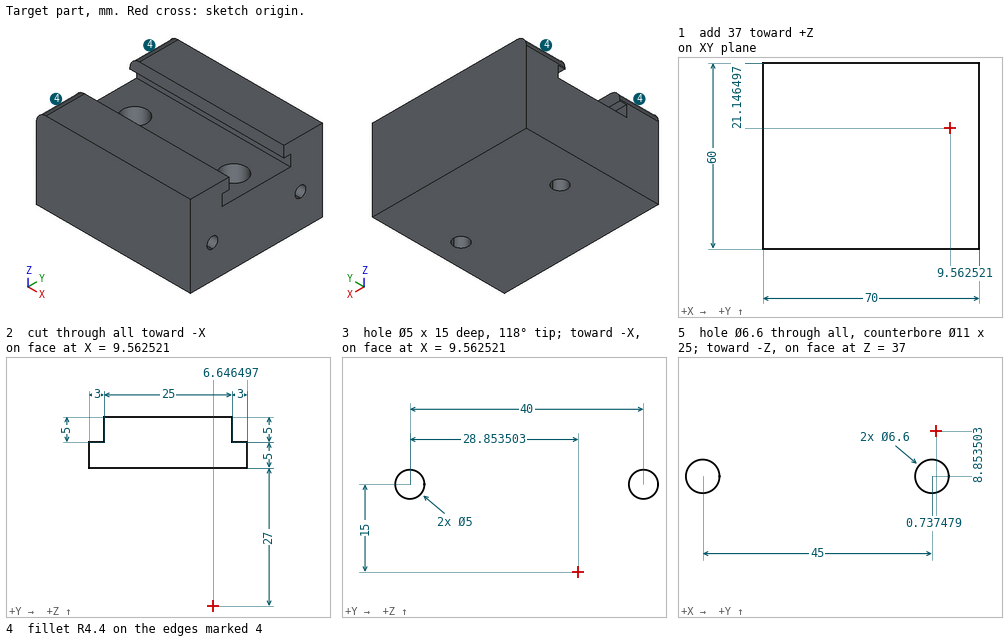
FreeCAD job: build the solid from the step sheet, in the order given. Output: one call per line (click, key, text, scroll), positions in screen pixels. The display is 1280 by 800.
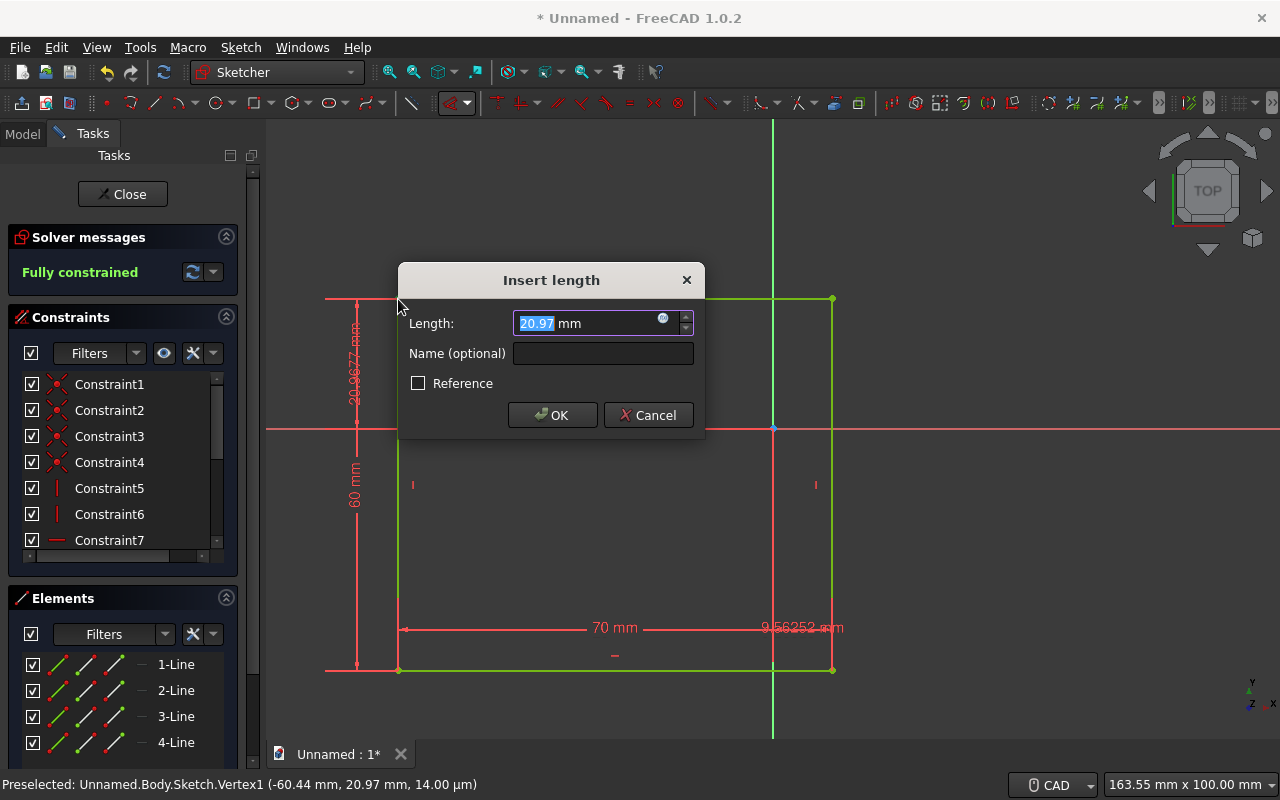
text(21.146497)
key(Return)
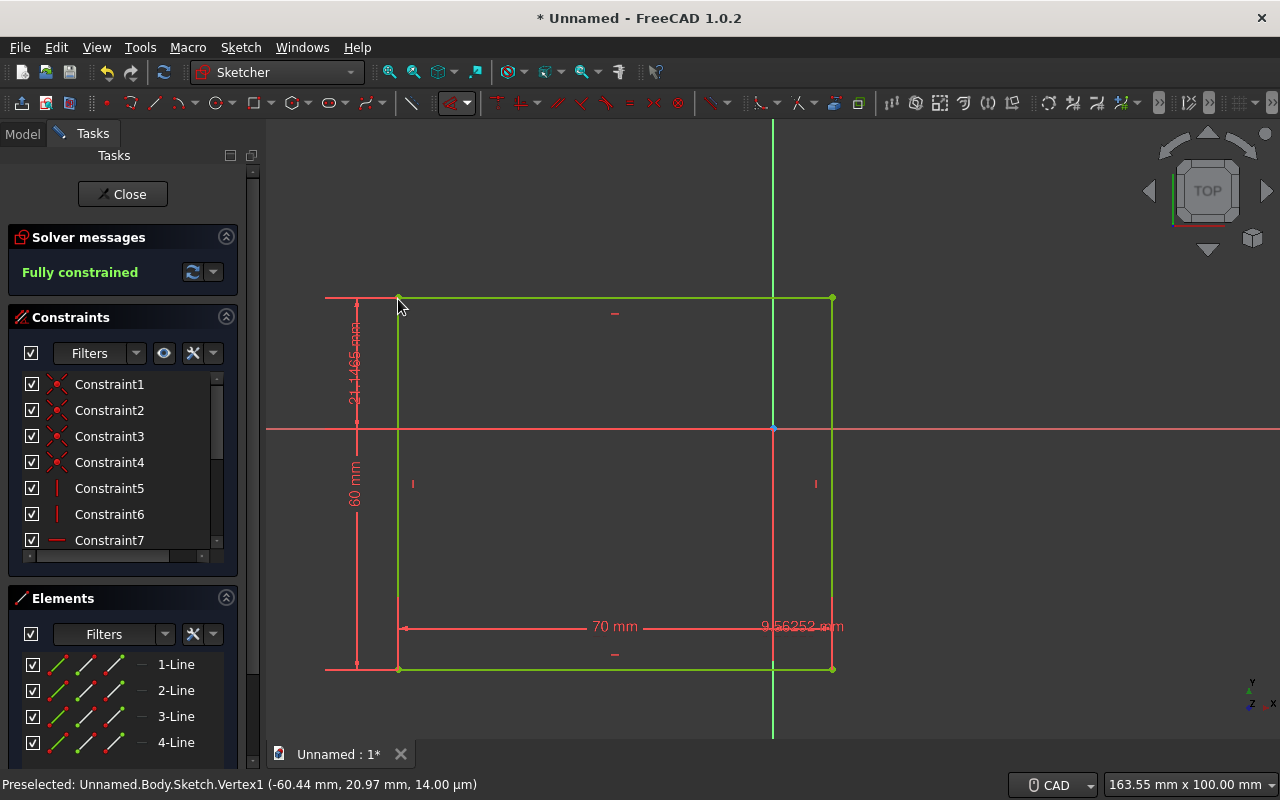
click(123, 194)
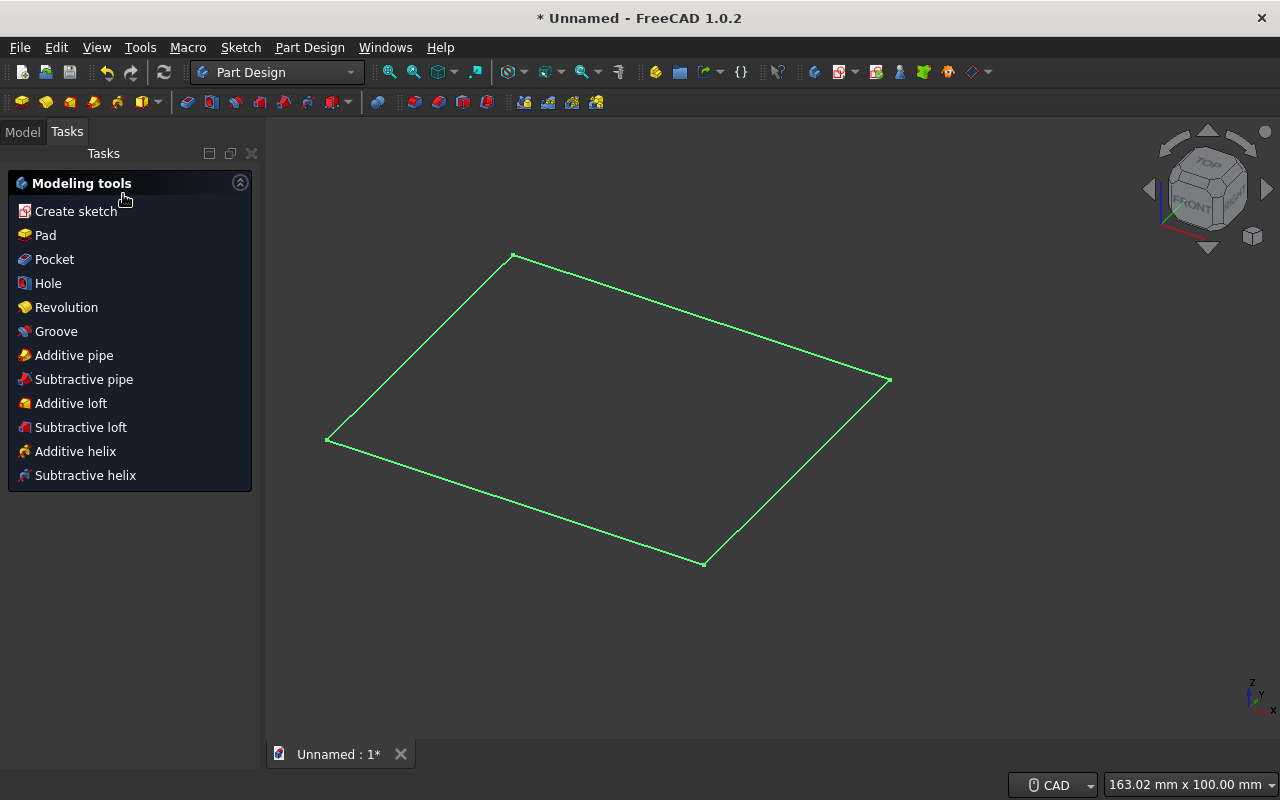
click(22, 102)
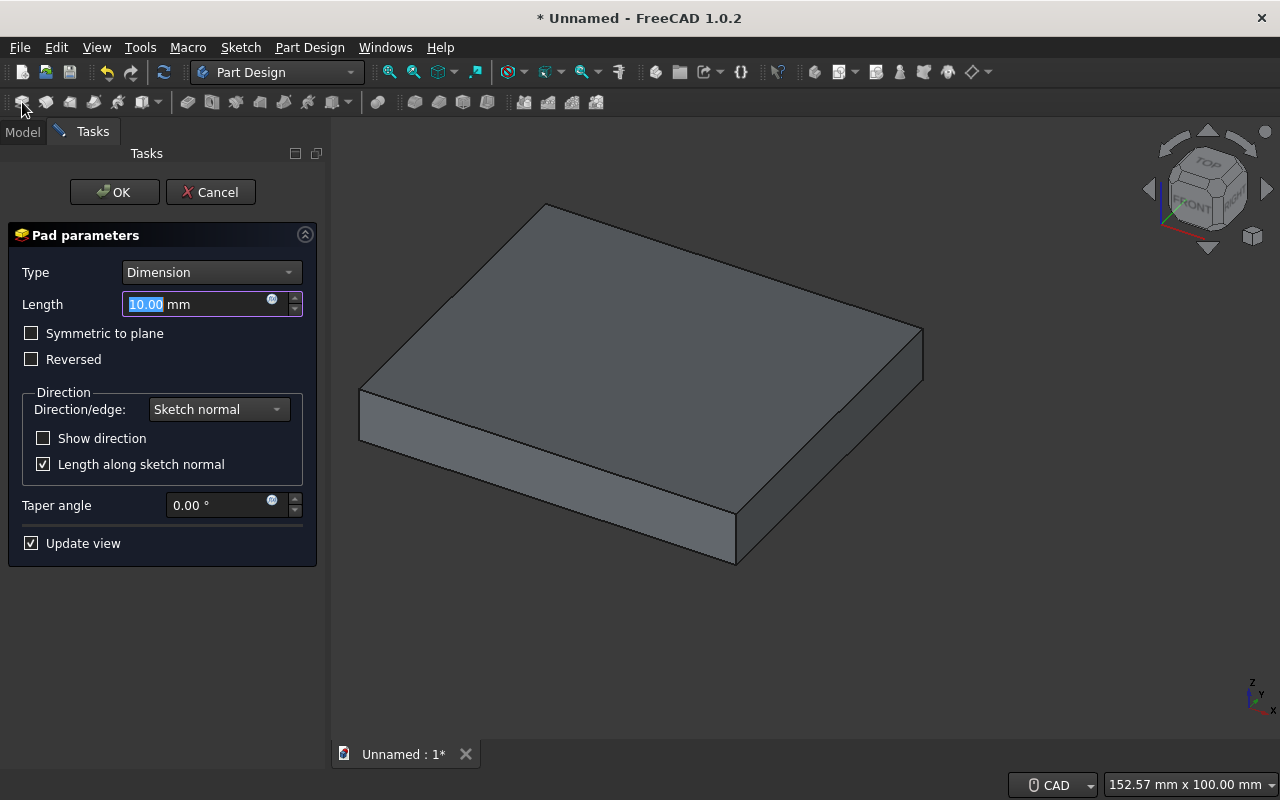
text(37)
key(Tab)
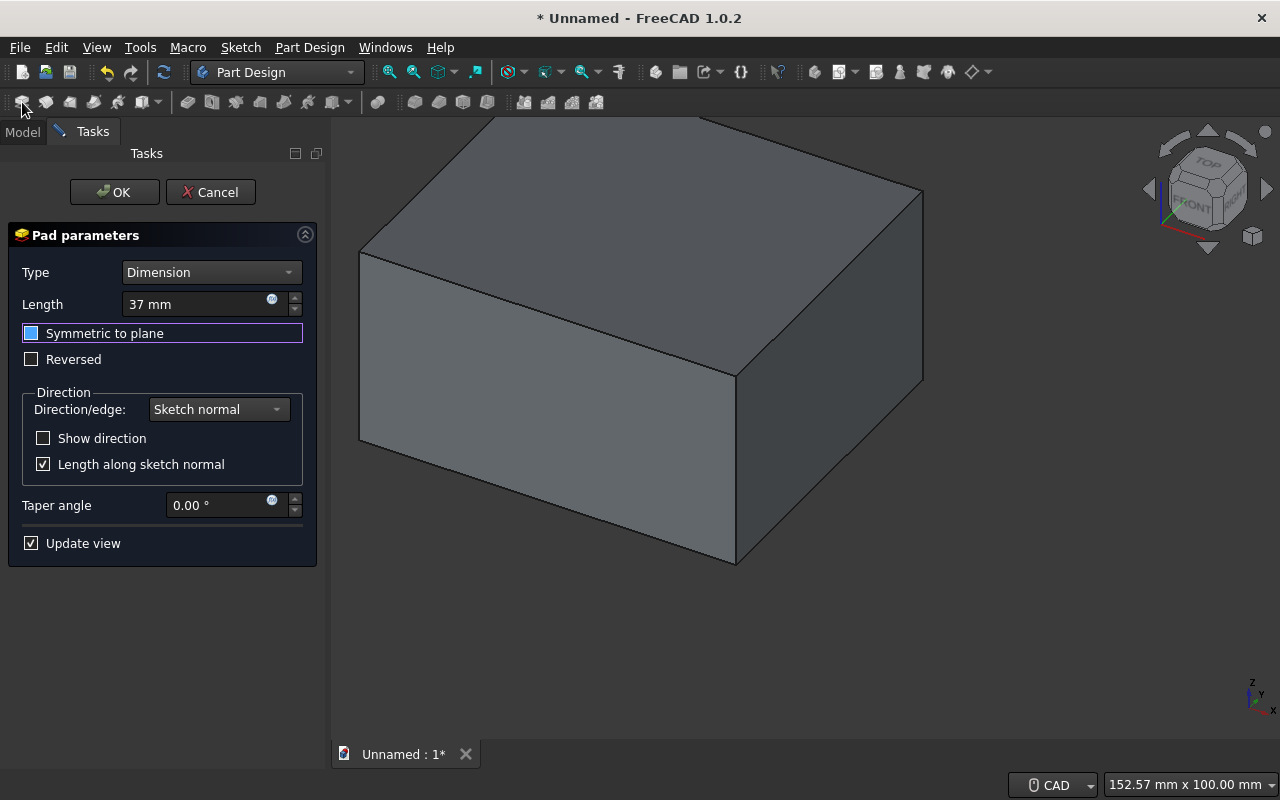
click(115, 192)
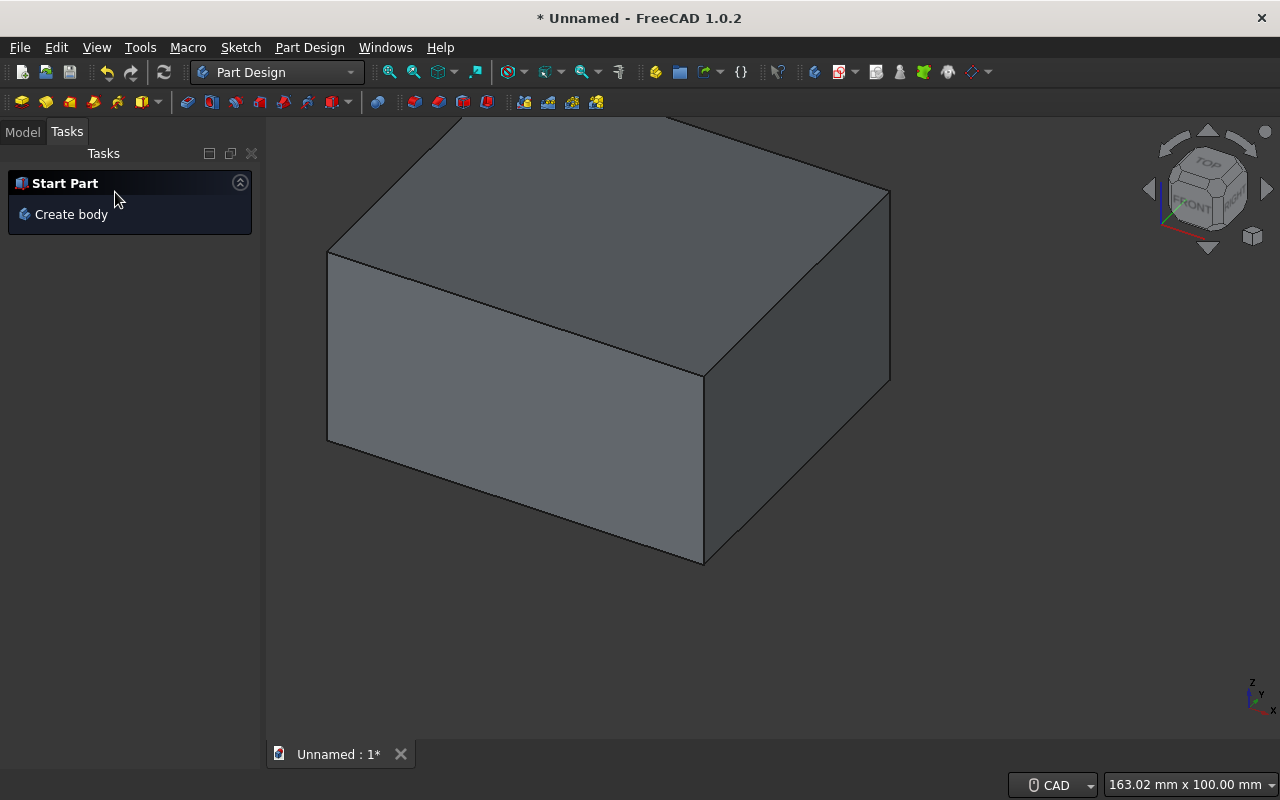
click(390, 72)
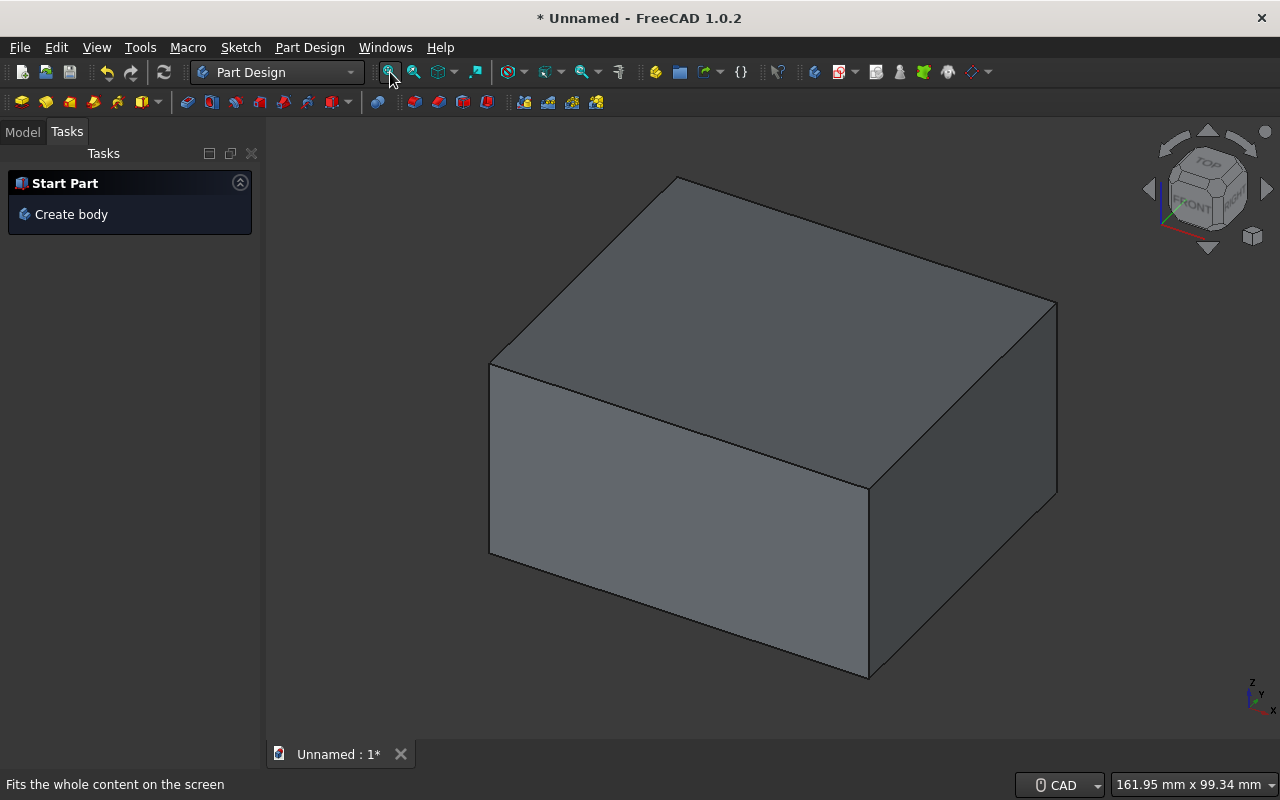
click(990, 463)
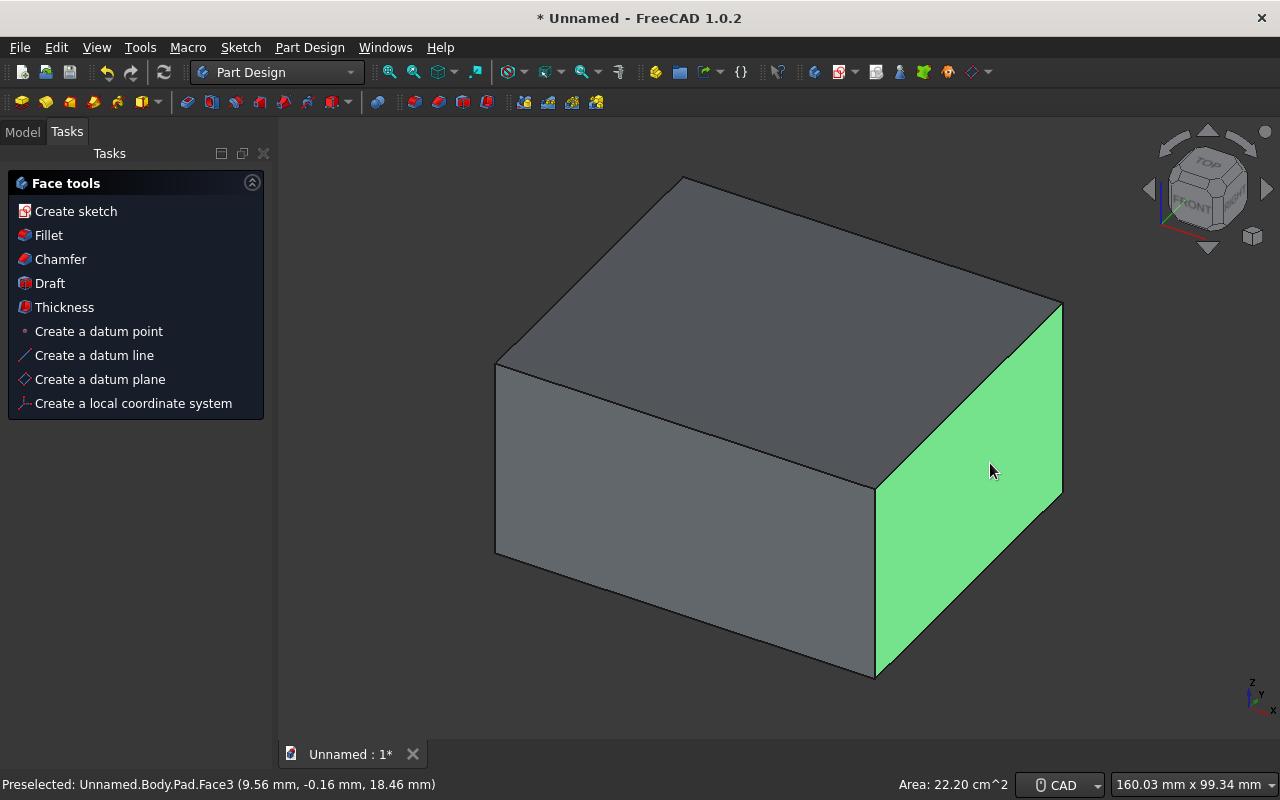
click(840, 72)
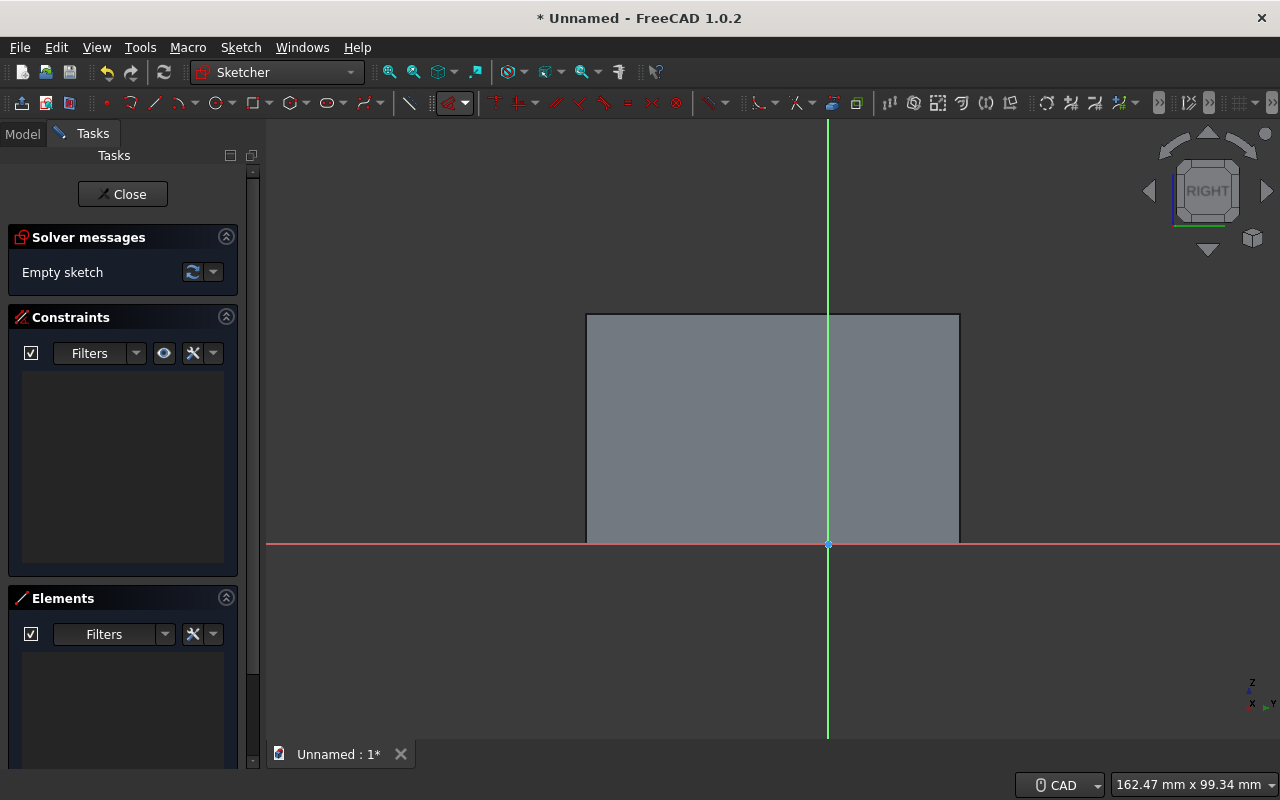
scroll(856, 429, up, 3)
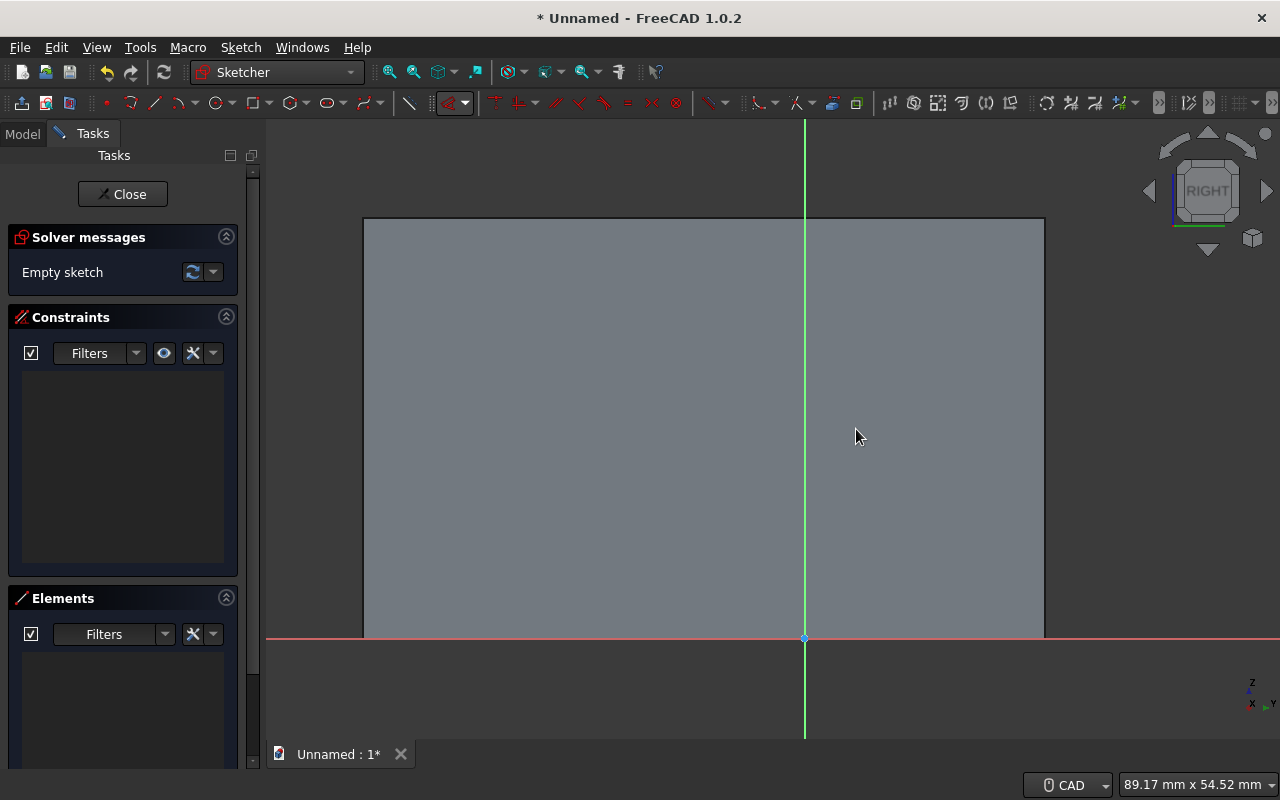
click(132, 104)